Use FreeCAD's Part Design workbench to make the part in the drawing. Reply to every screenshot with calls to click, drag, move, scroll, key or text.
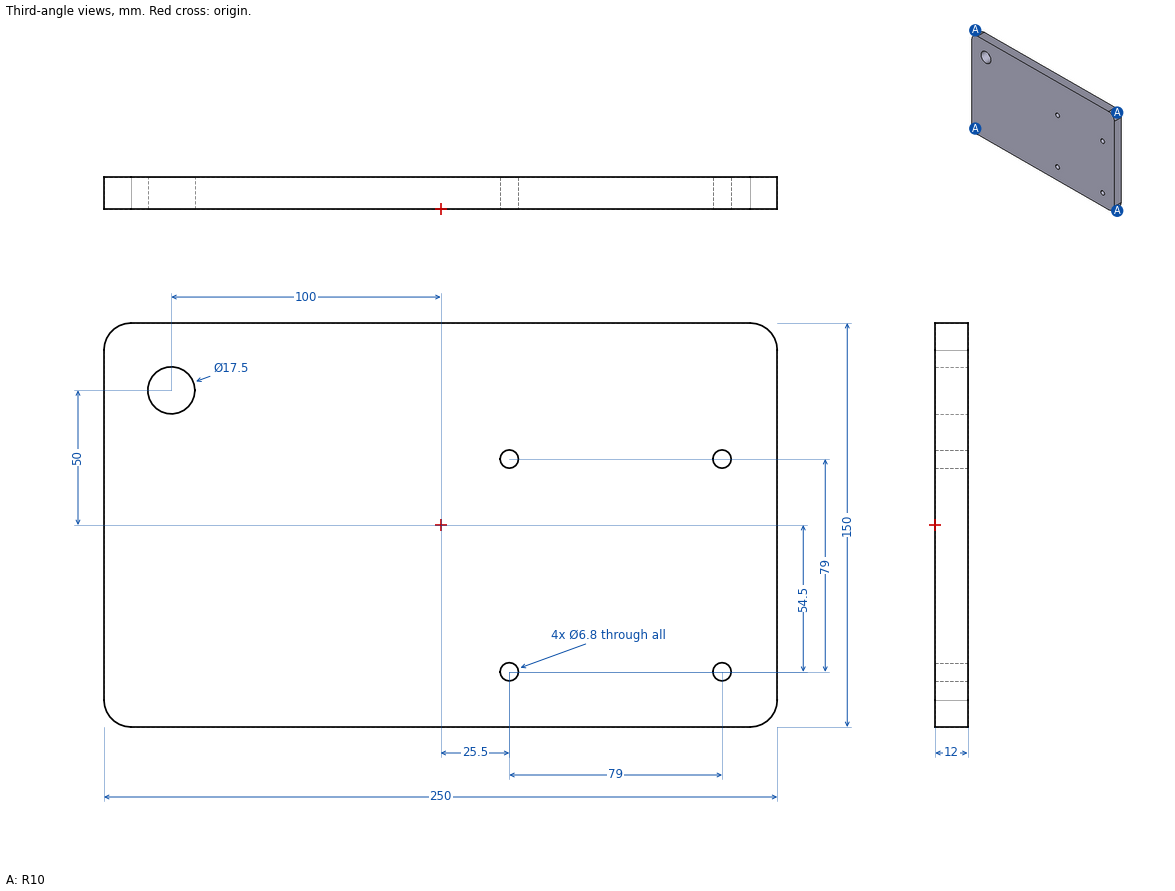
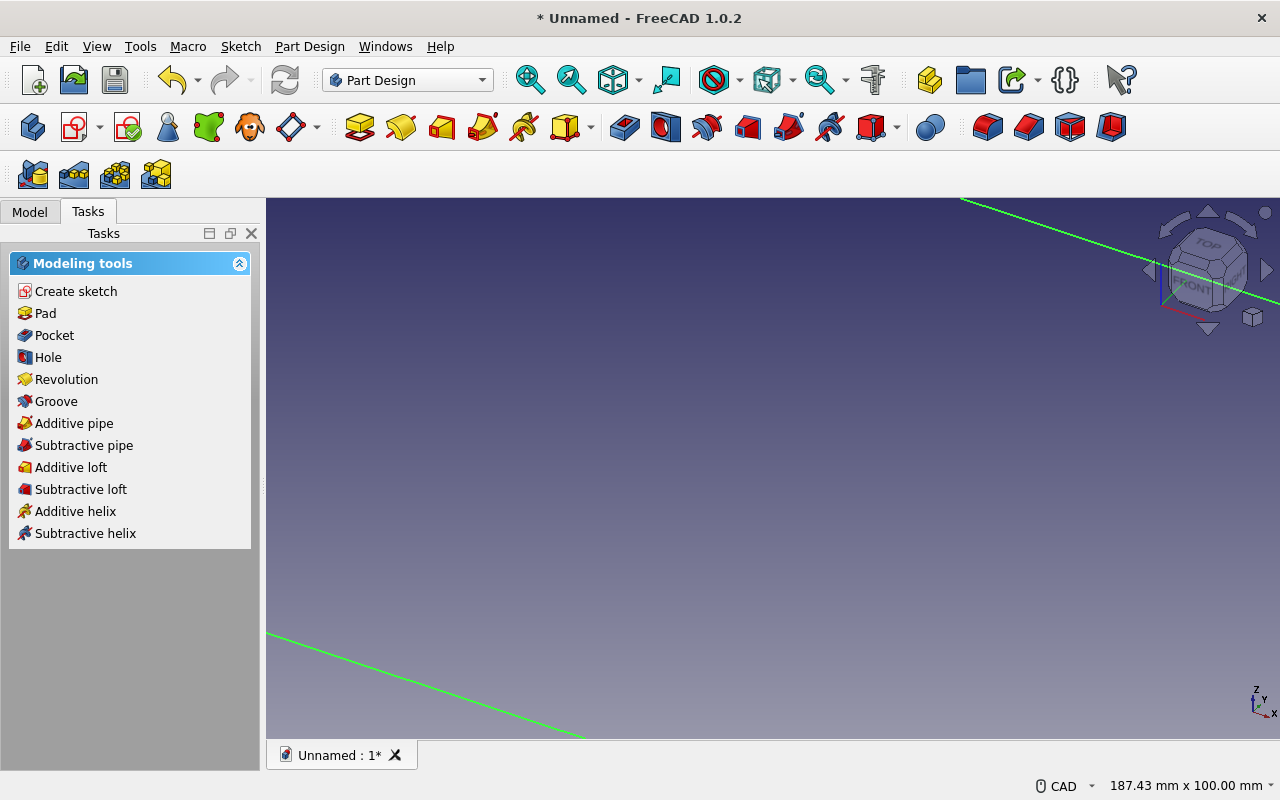
click(360, 128)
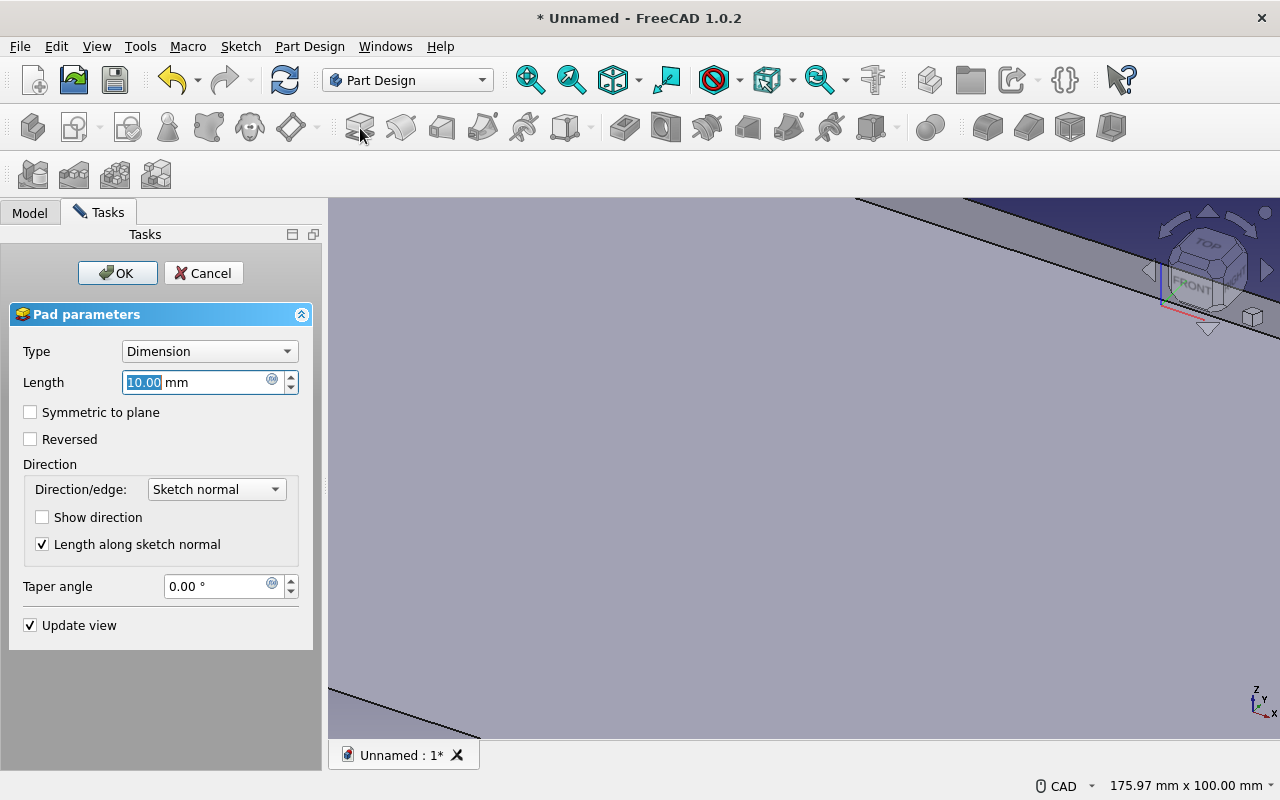
text(12)
key(Tab)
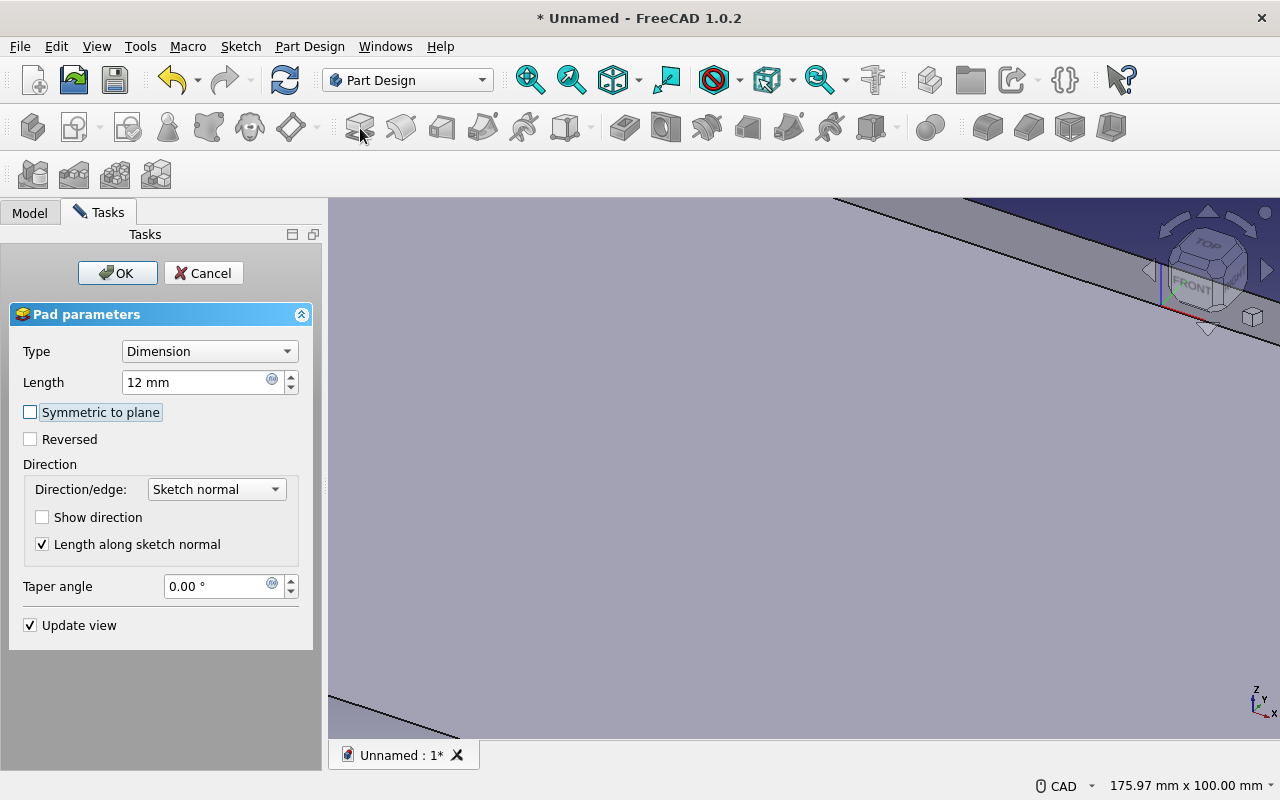
click(31, 439)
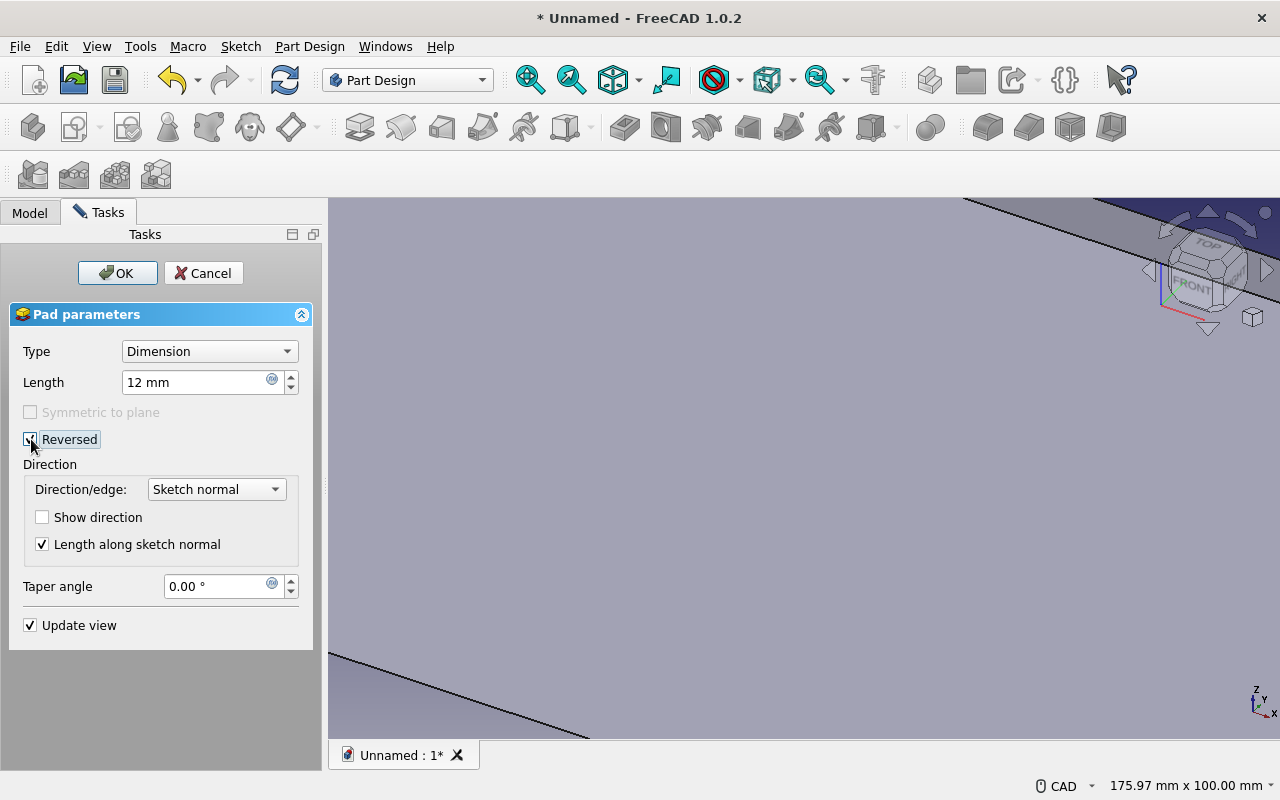
click(118, 273)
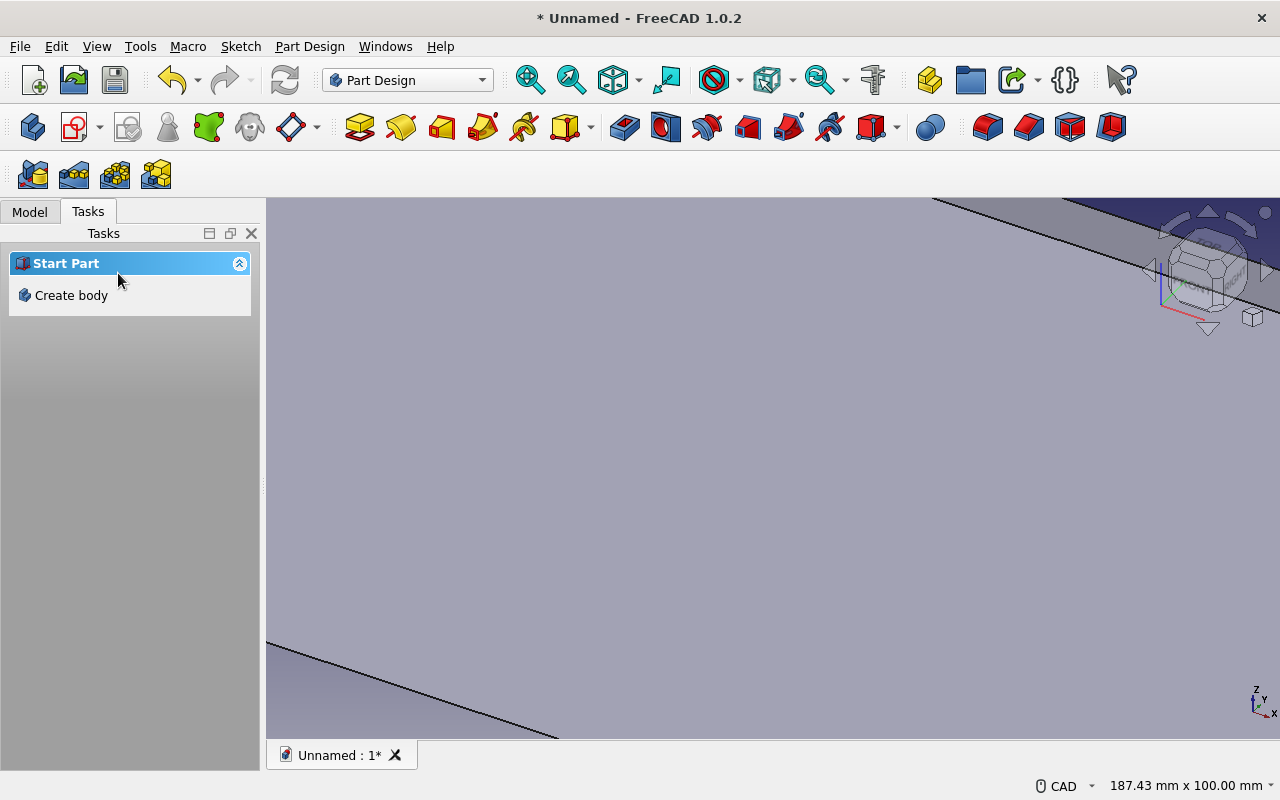
click(531, 80)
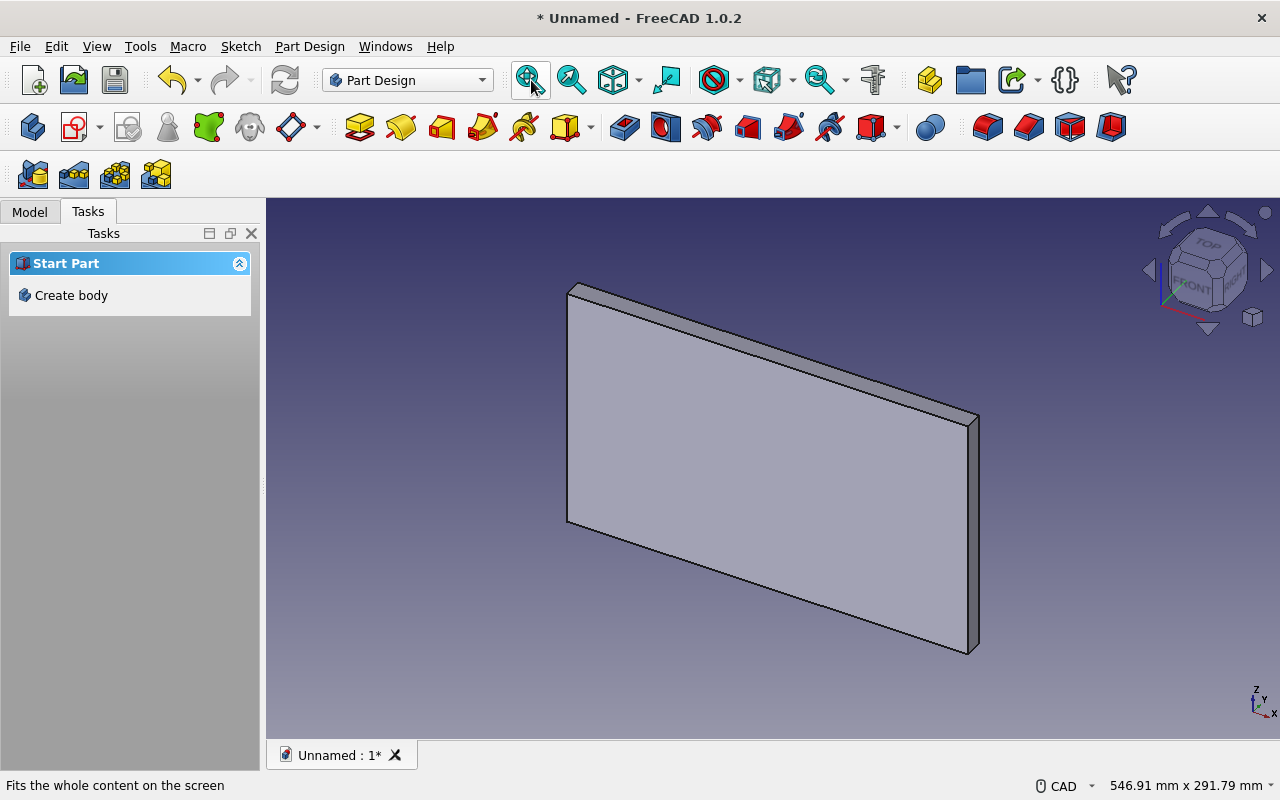
click(825, 492)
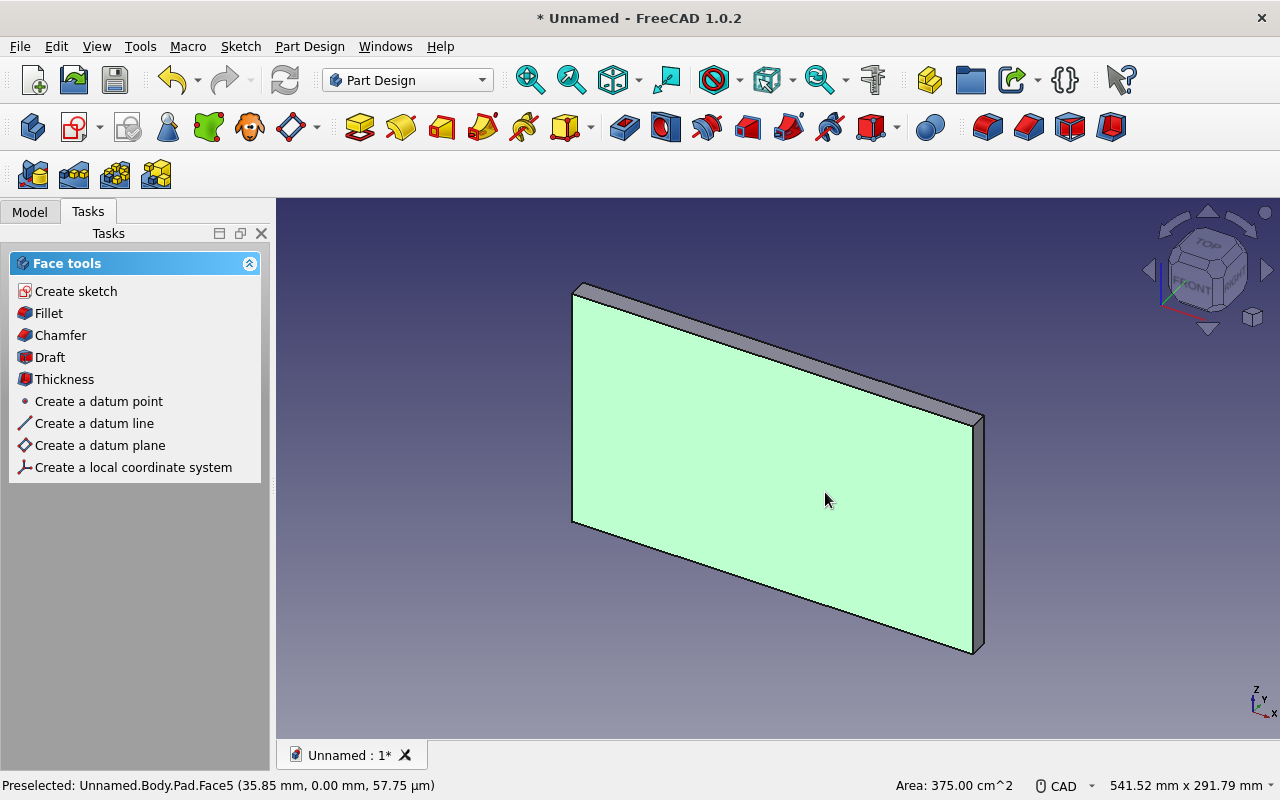
click(74, 128)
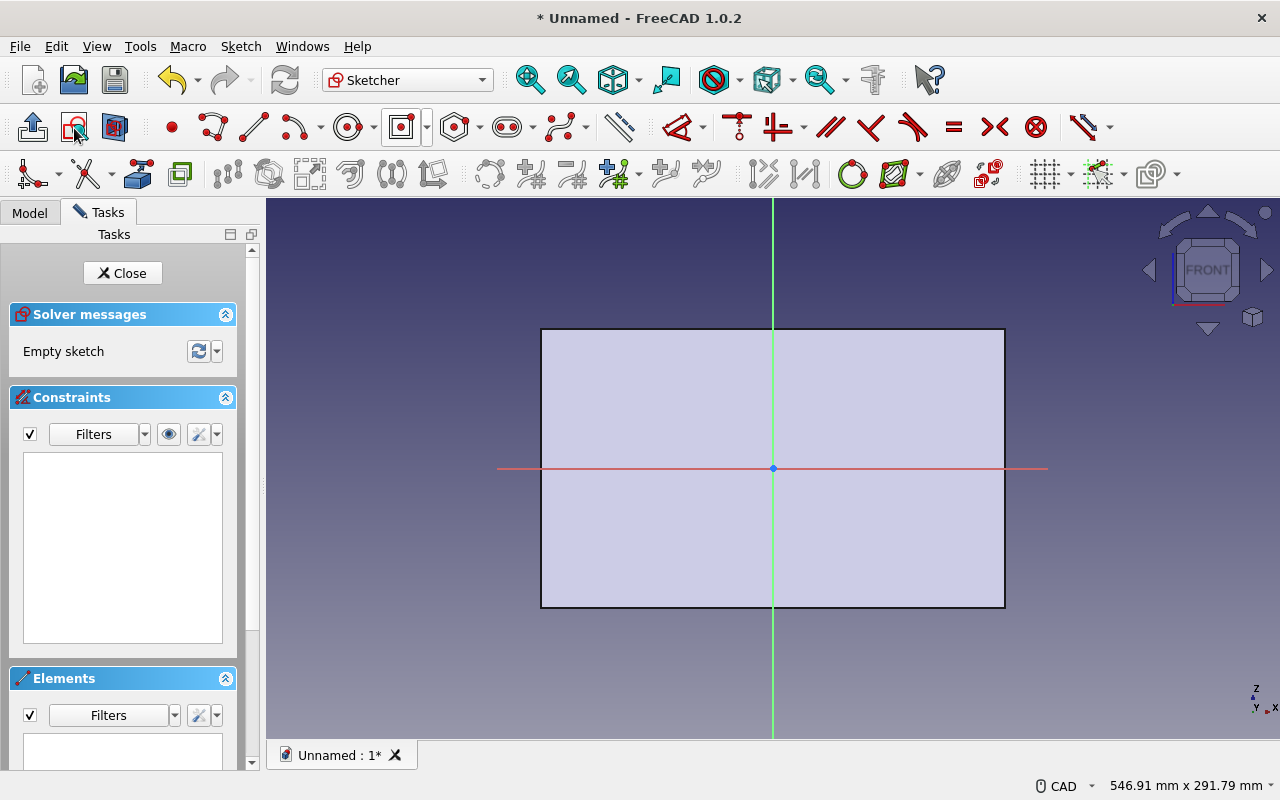
scroll(576, 367, up, 12)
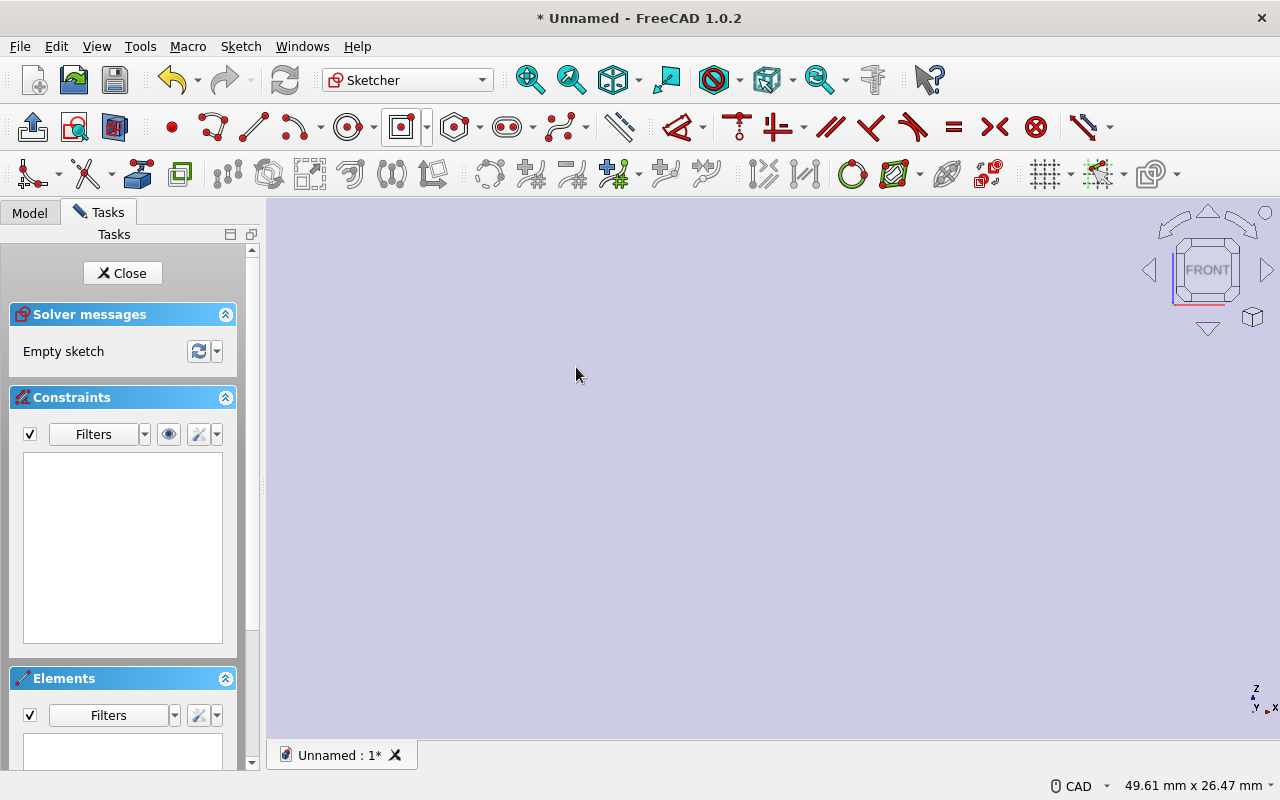
click(348, 128)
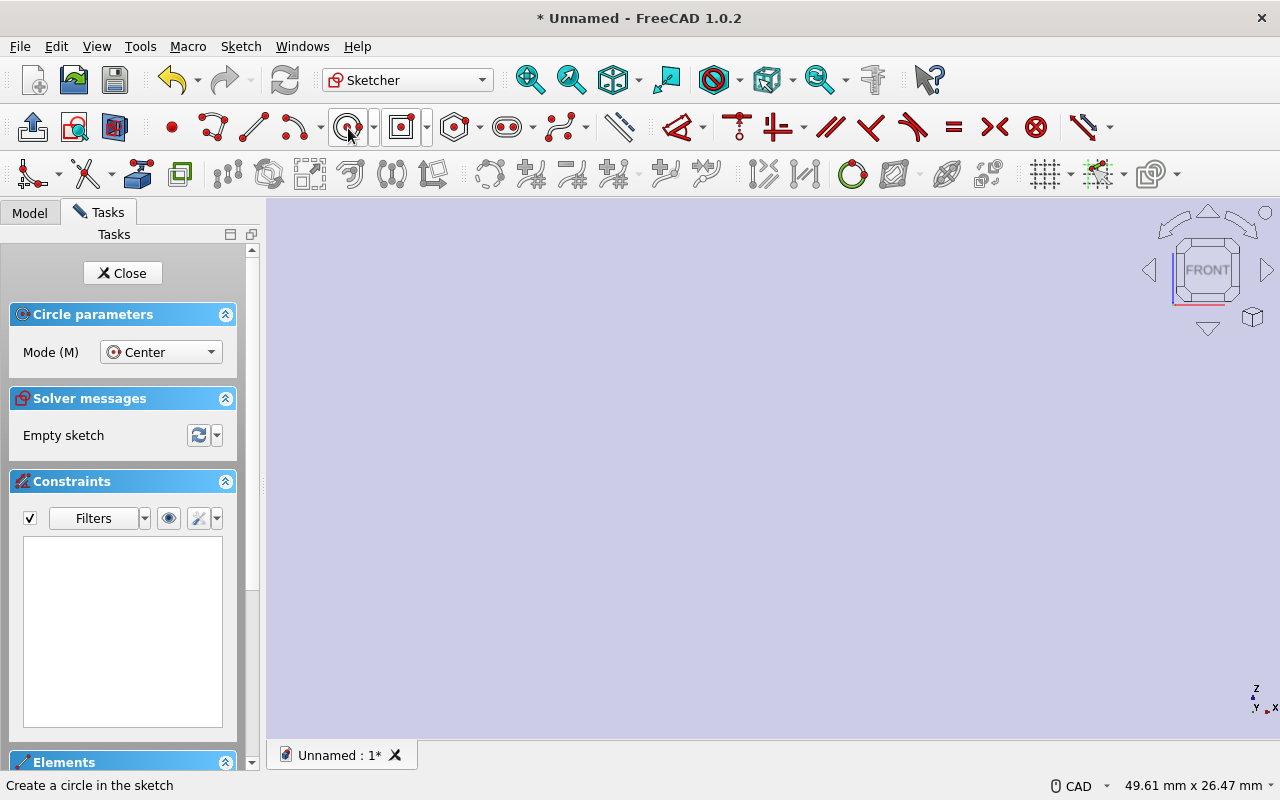
click(701, 461)
move(827, 334)